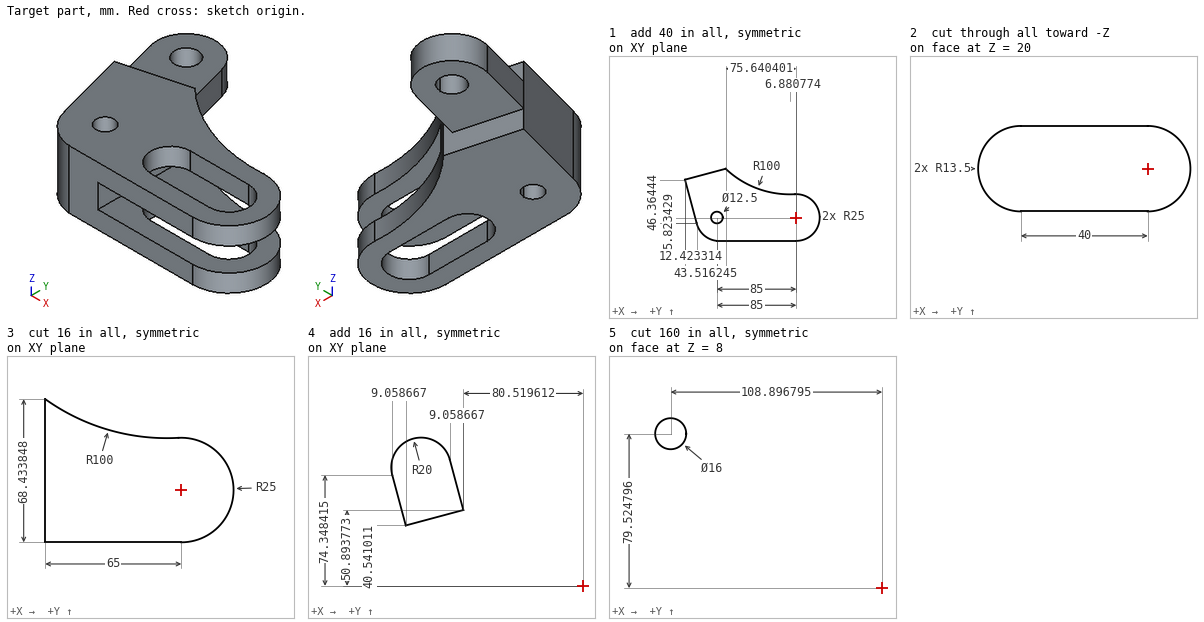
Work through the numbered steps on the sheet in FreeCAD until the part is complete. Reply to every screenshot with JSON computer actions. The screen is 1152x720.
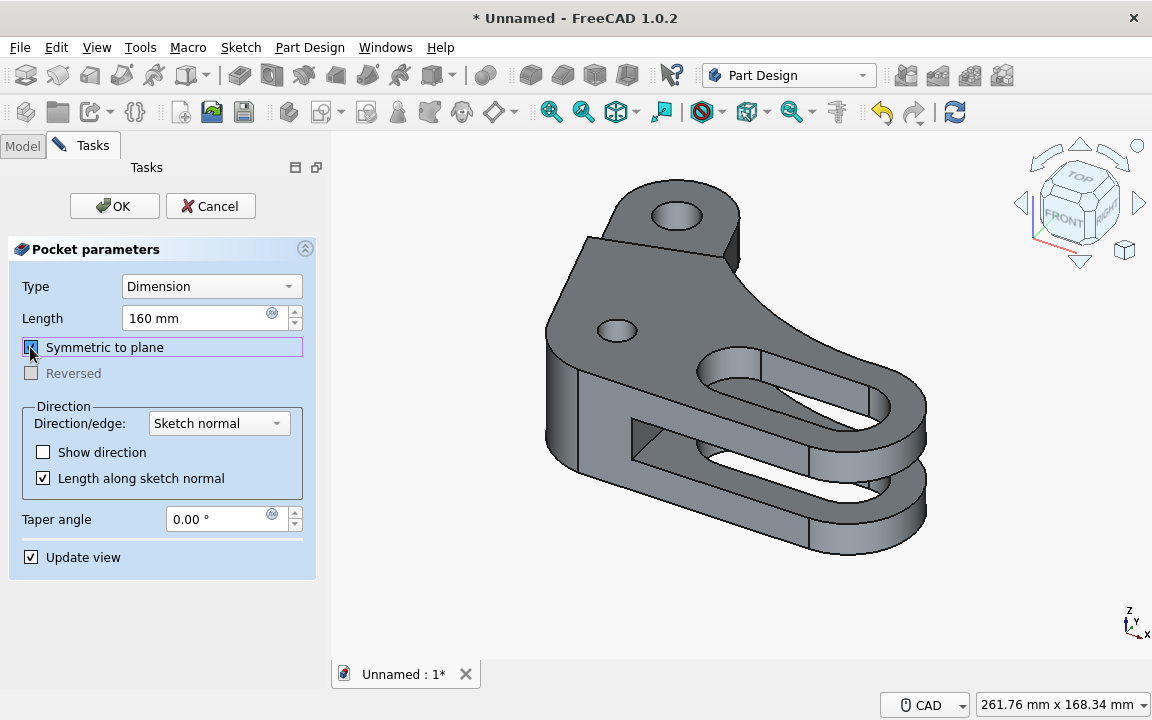
{"action": "left_click", "coordinate": [115, 206]}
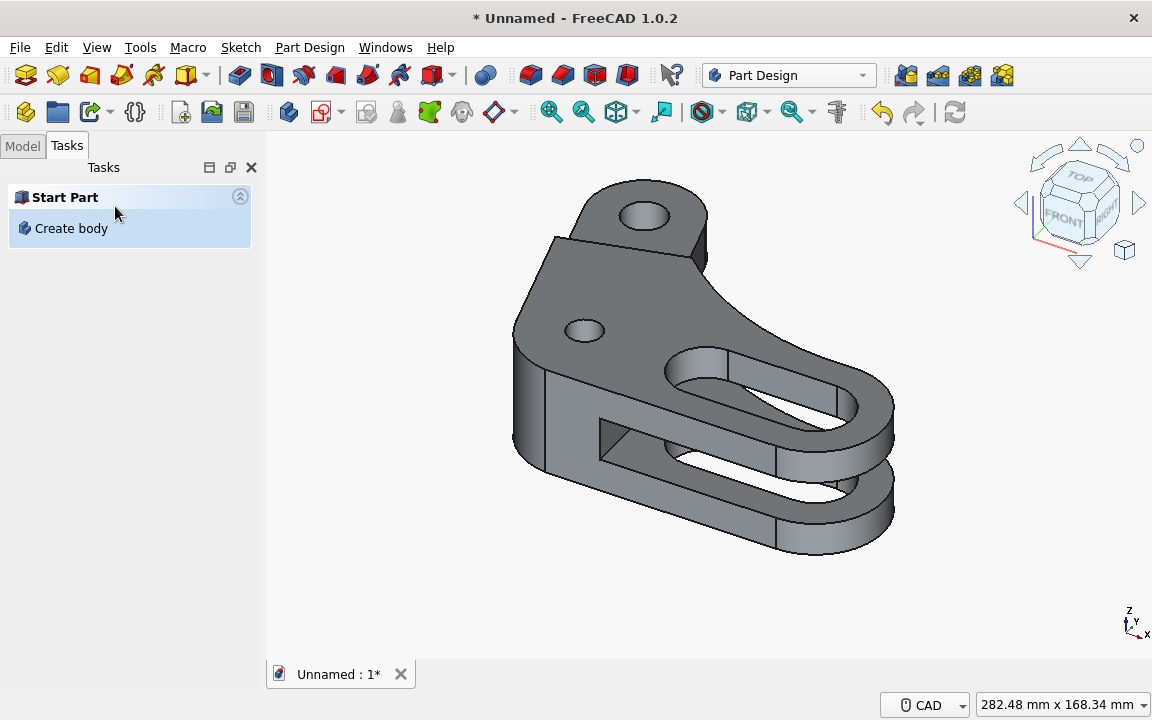
{"action": "key", "text": "0"}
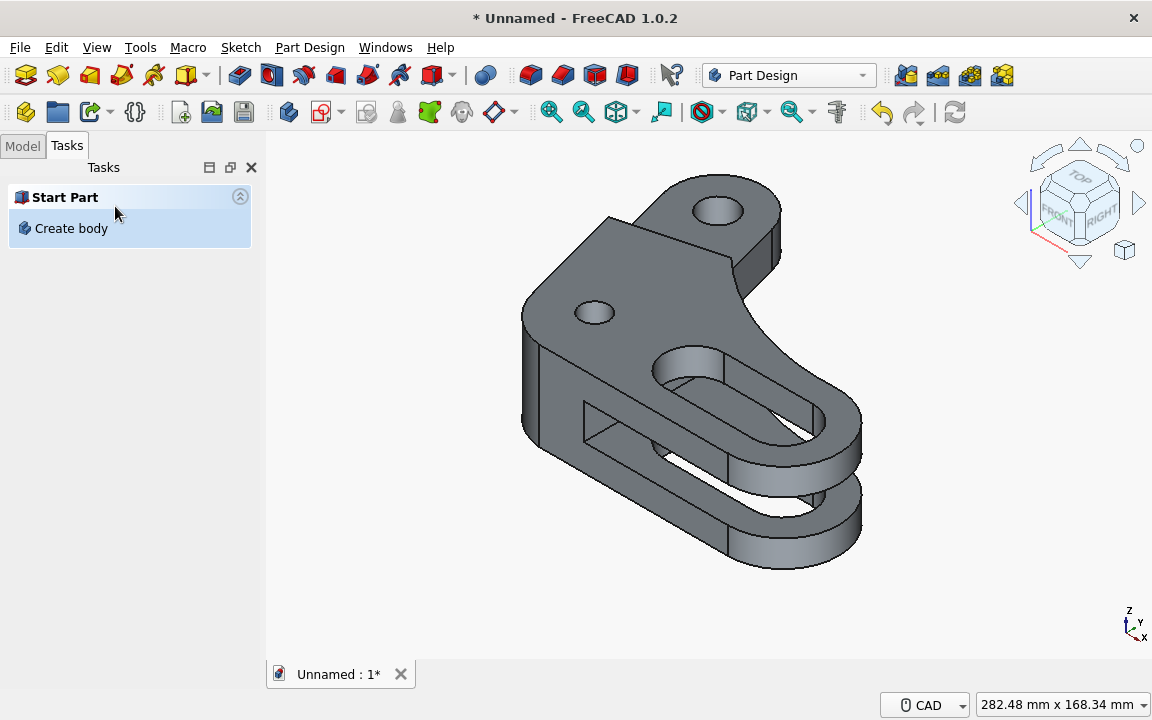
{"action": "left_click", "coordinate": [552, 112]}